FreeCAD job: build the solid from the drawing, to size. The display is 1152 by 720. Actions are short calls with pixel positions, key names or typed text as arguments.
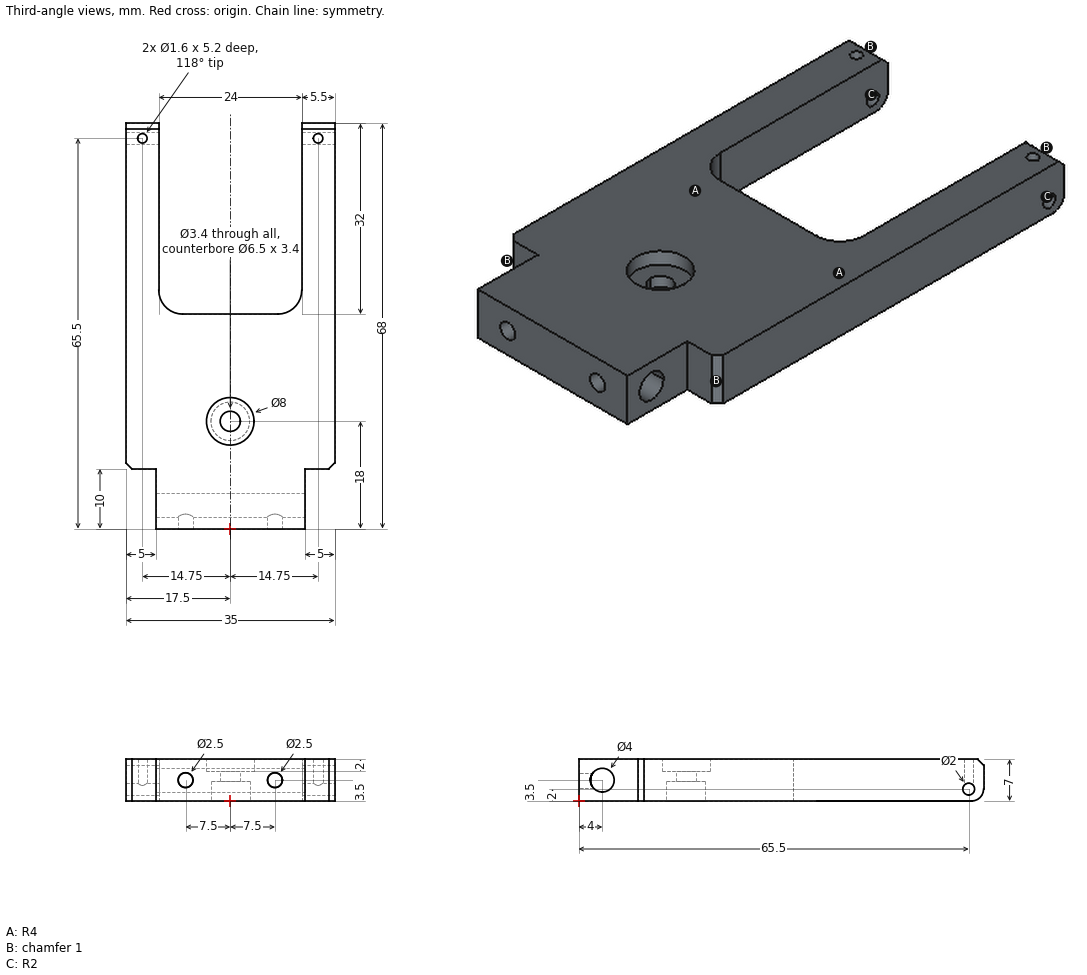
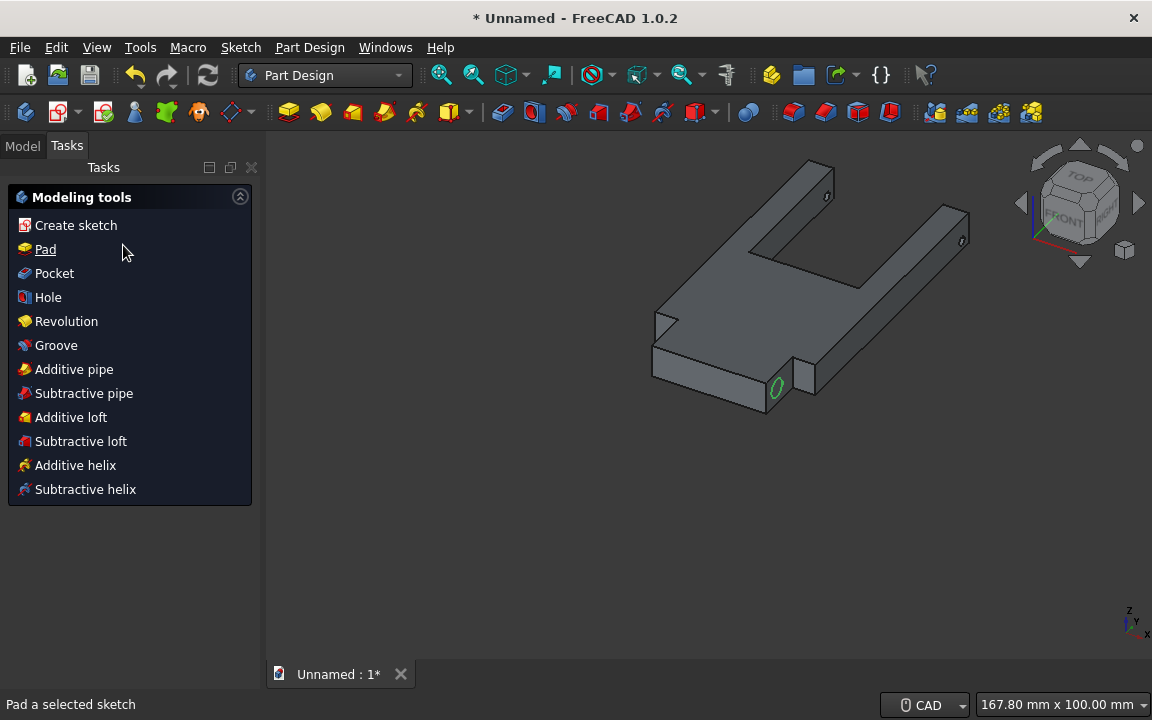
click(504, 112)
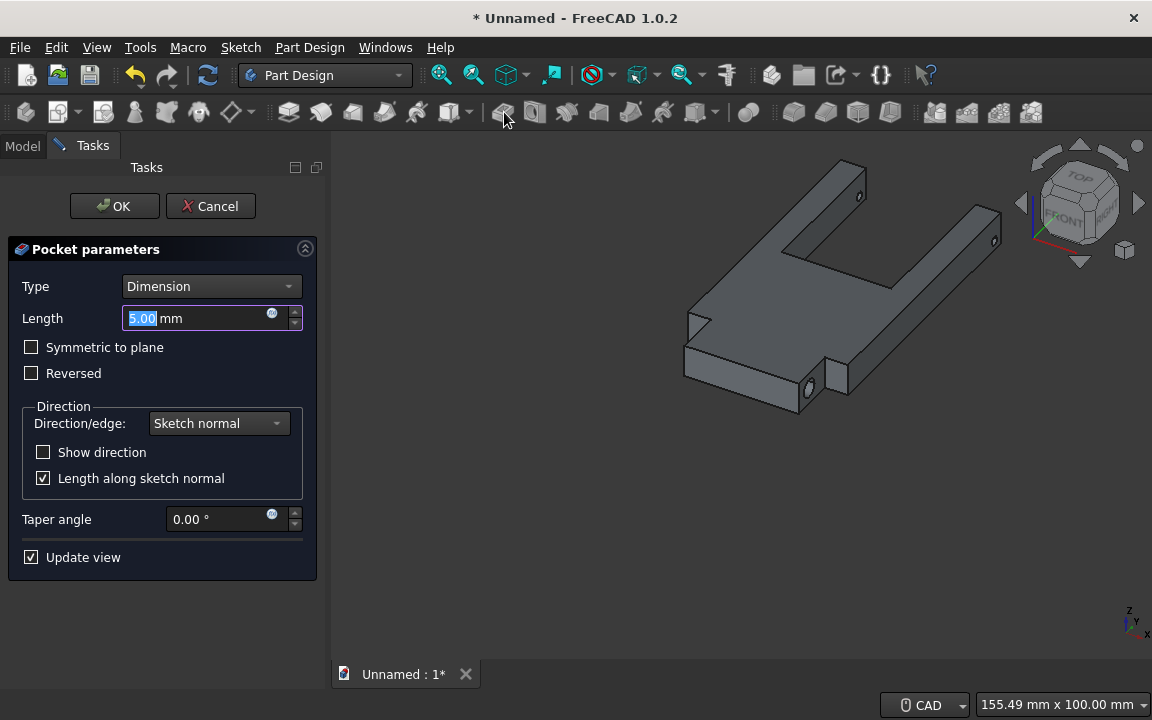
click(212, 286)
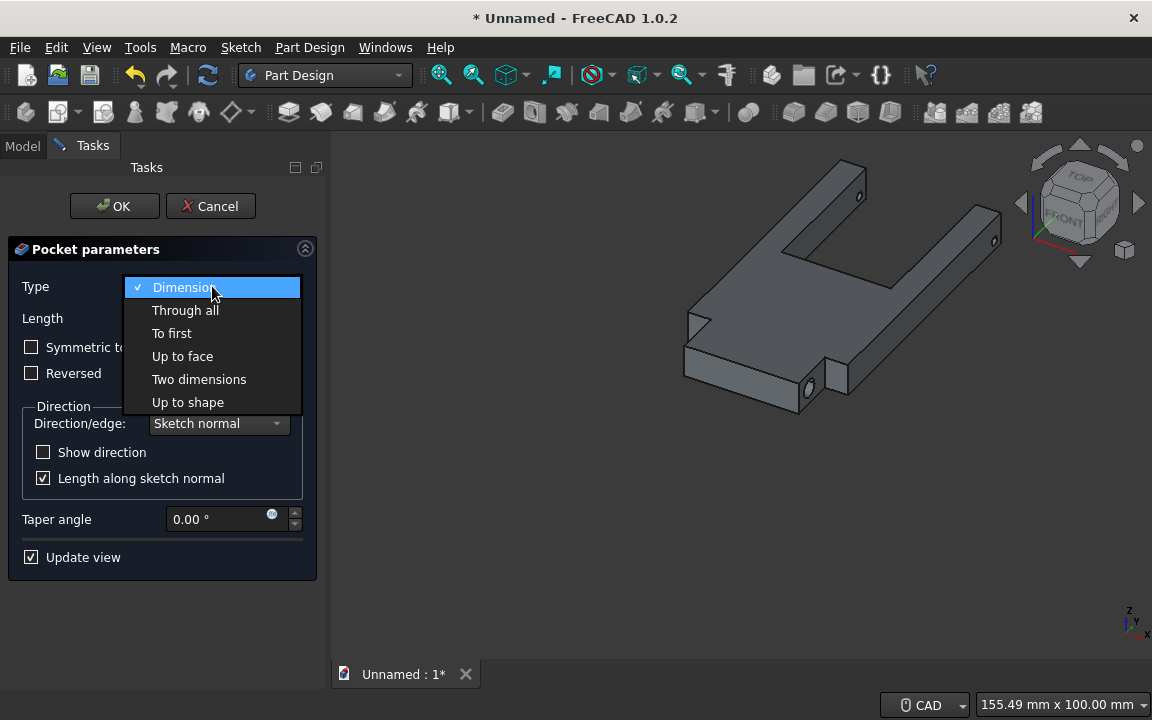
click(212, 310)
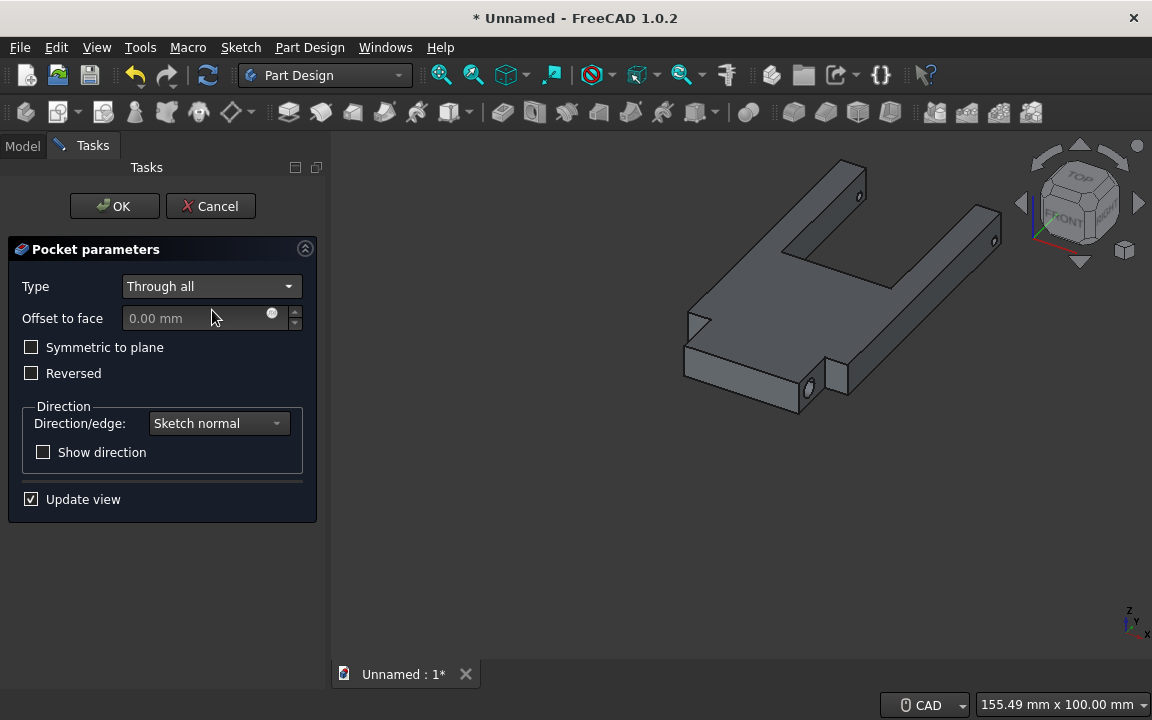
click(115, 206)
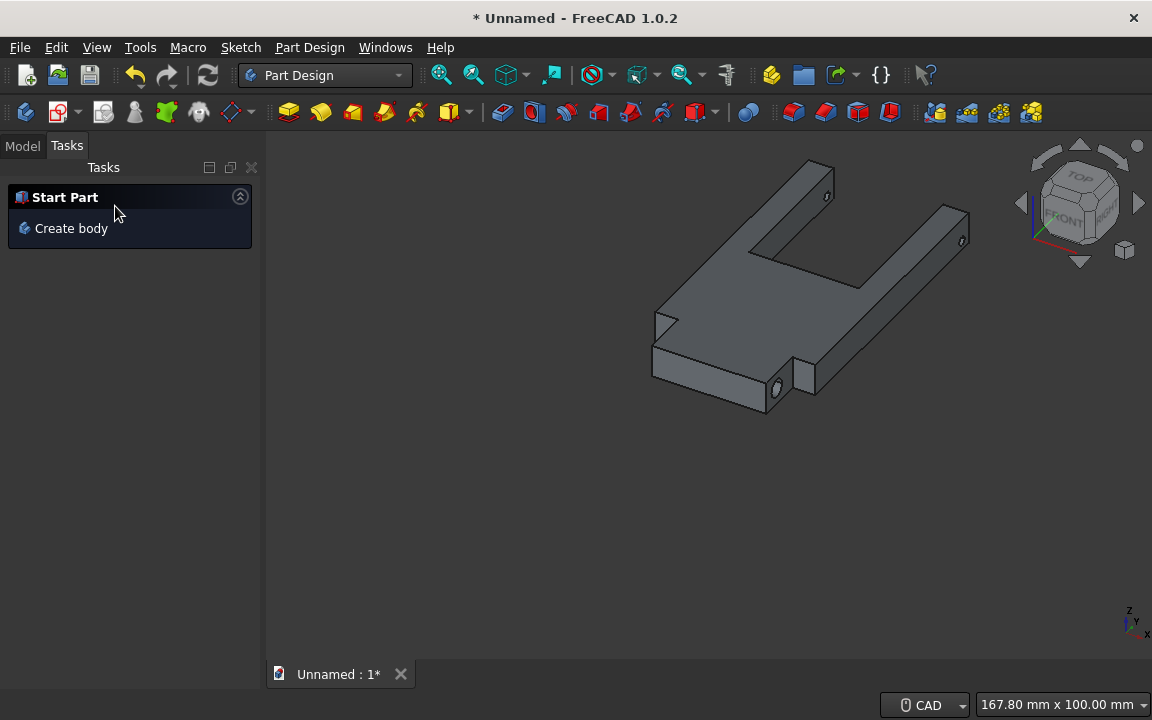
click(742, 390)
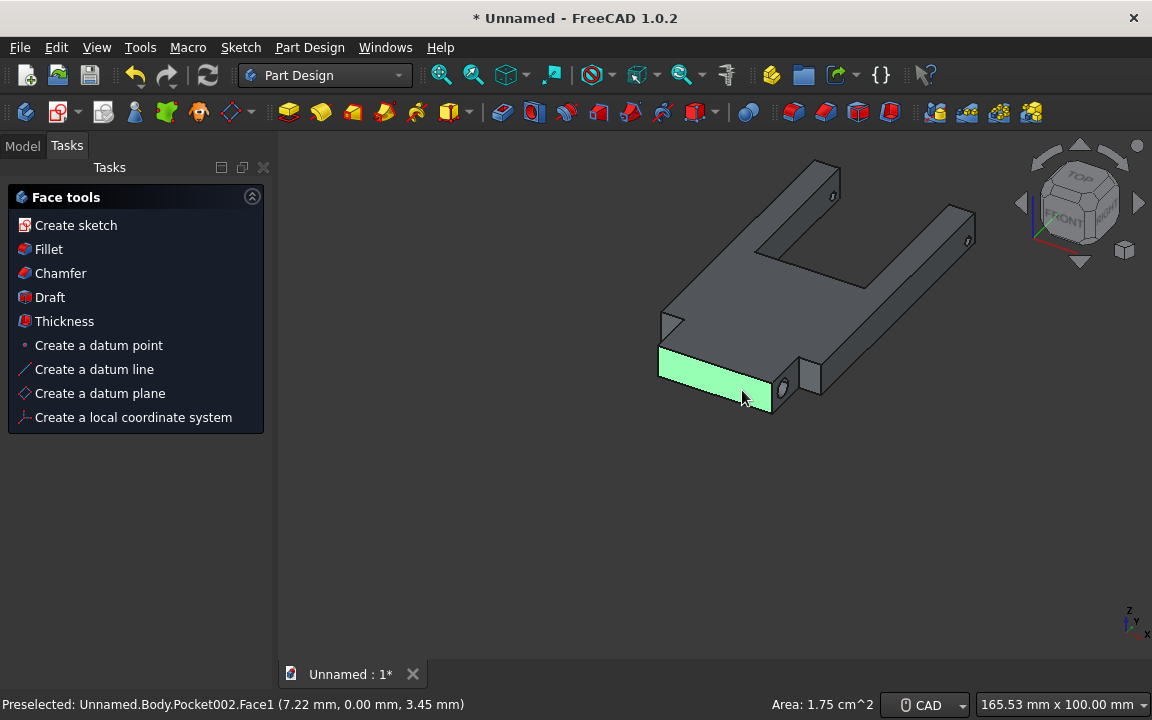
click(58, 112)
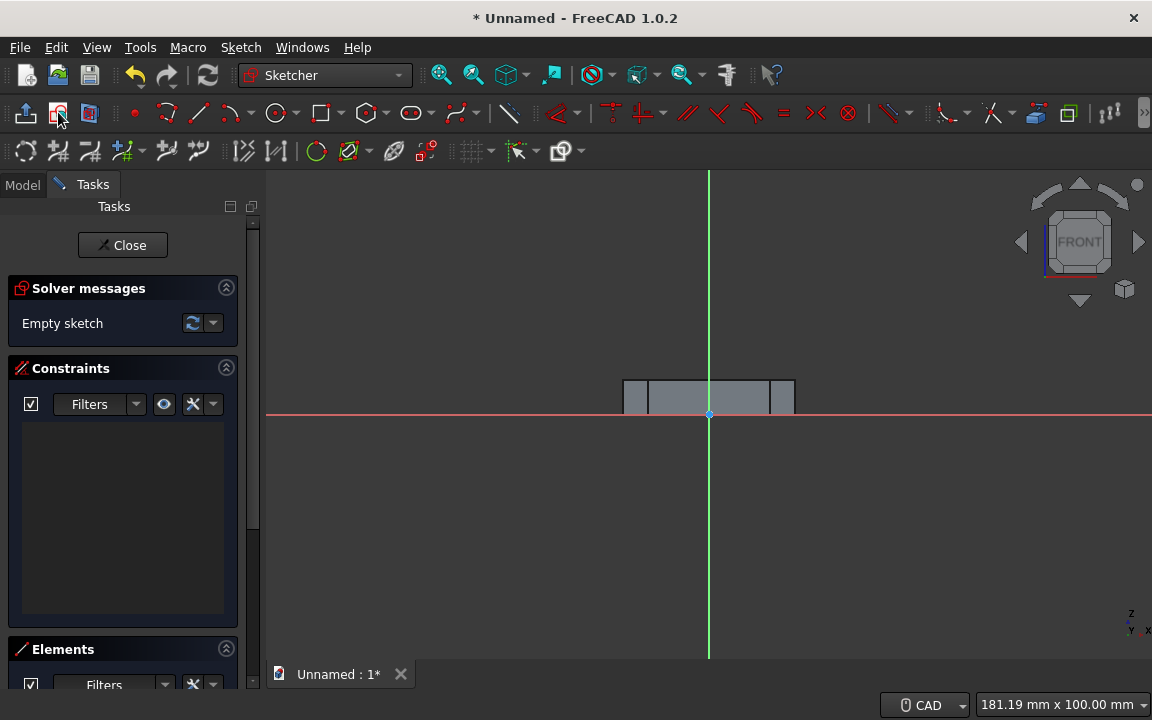
scroll(751, 396, up, 15)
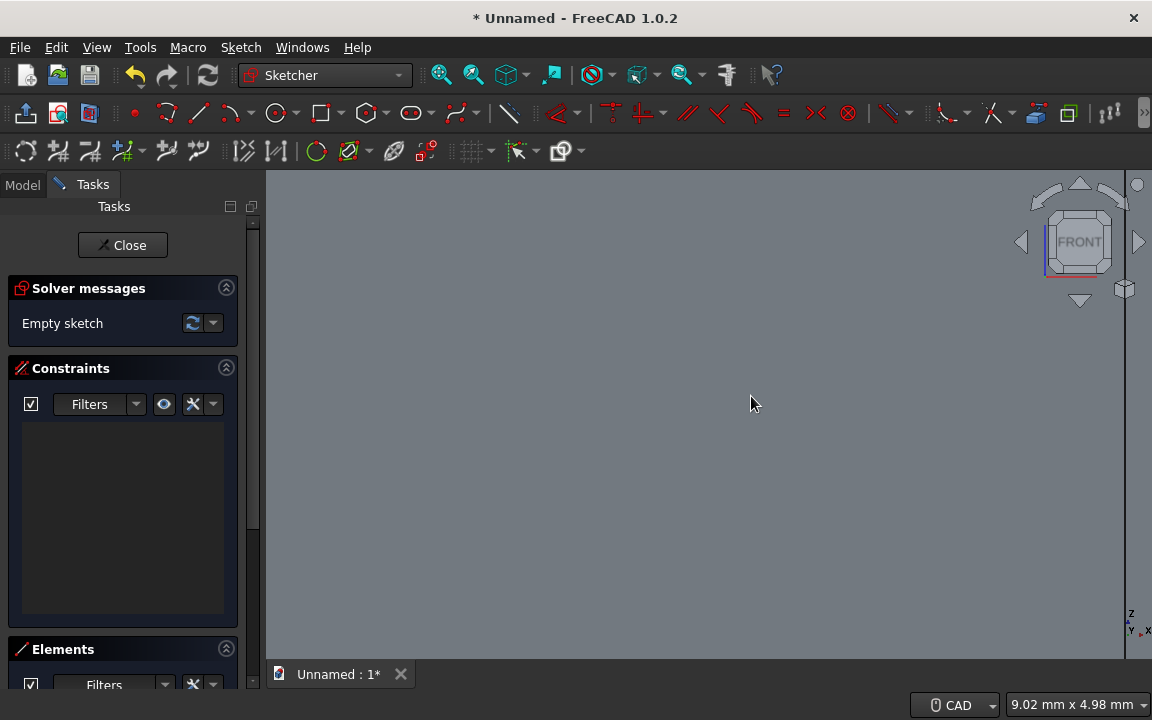
key(g)
key(c)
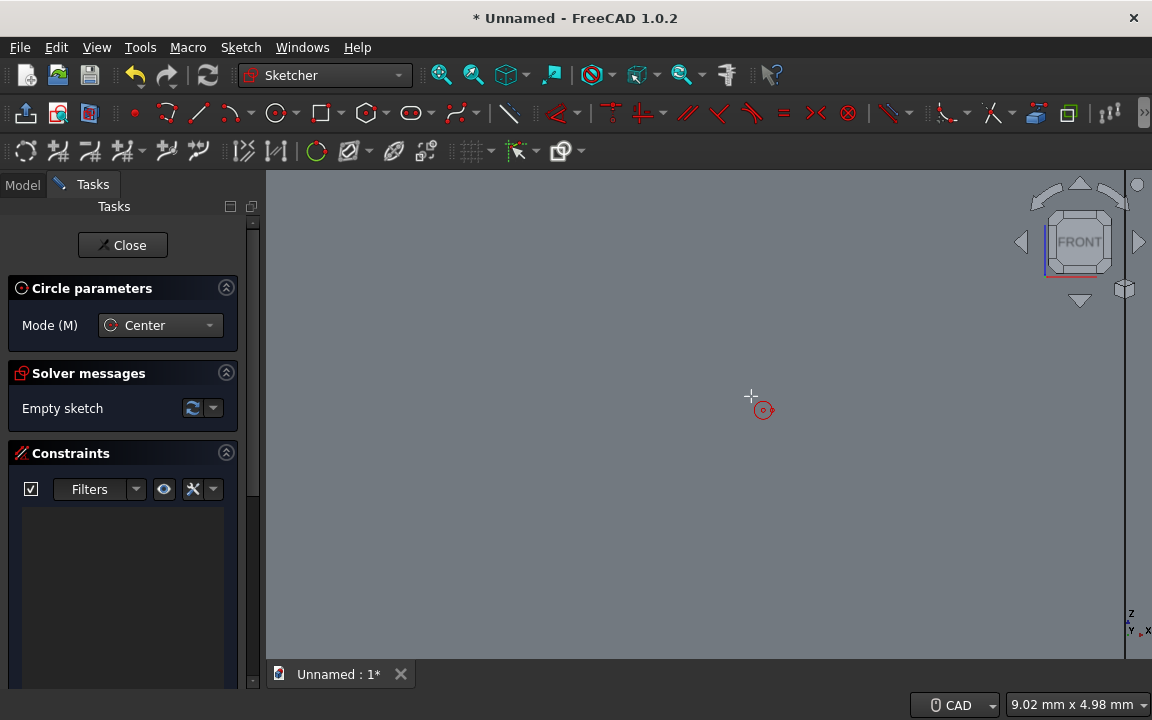
click(634, 415)
move(720, 328)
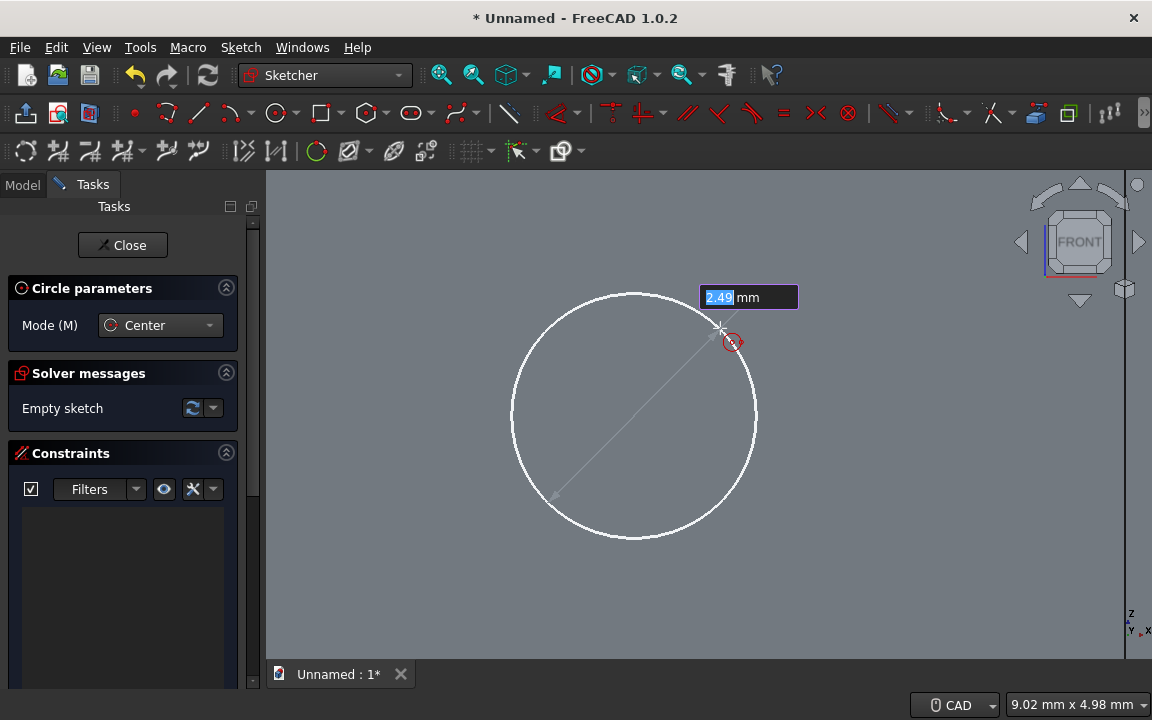
text(2.5)
key(Return)
key(Escape)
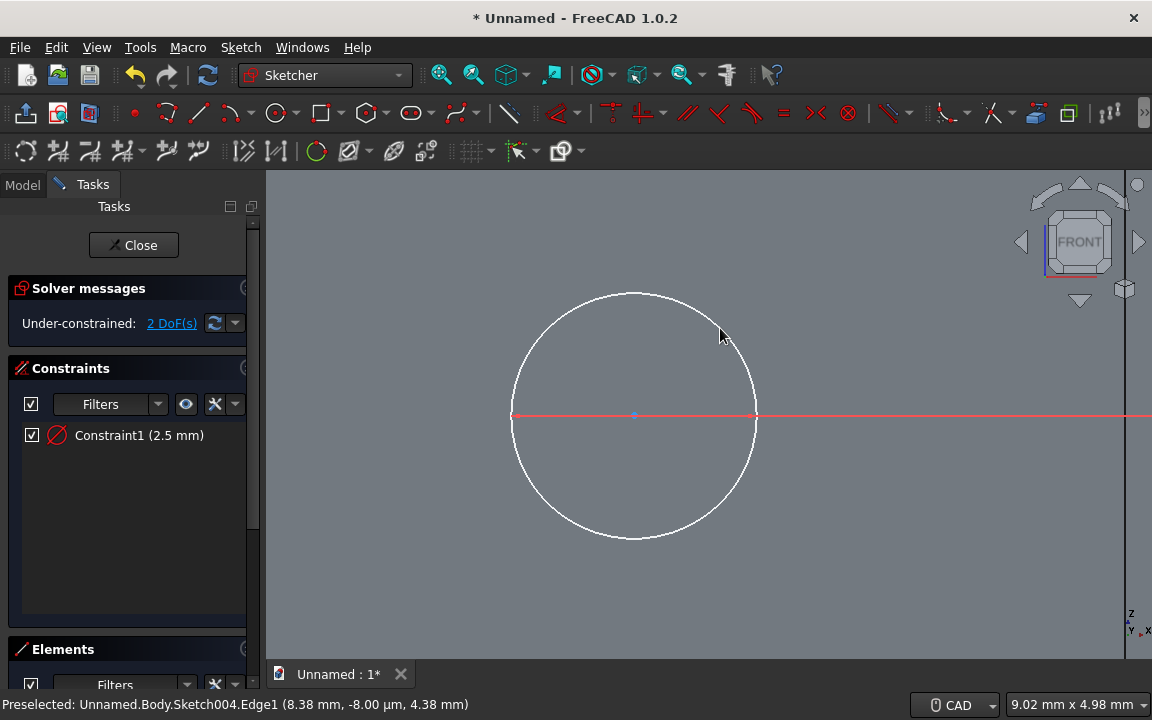
key(d)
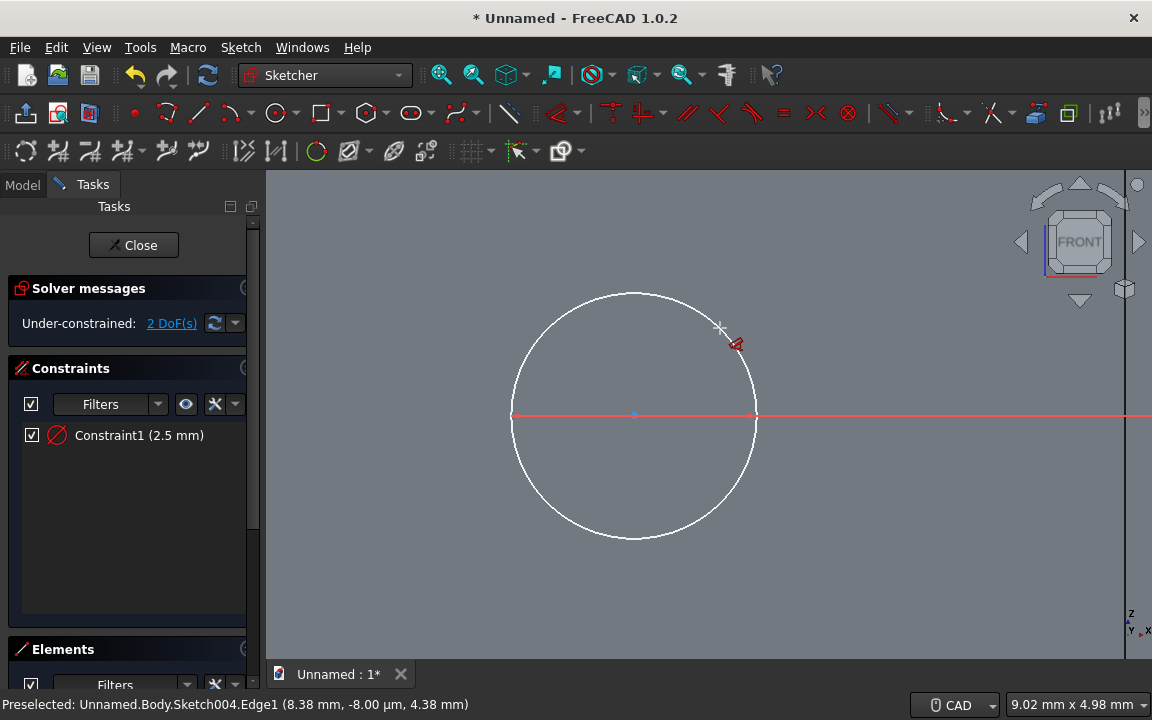
click(634, 416)
click(464, 382)